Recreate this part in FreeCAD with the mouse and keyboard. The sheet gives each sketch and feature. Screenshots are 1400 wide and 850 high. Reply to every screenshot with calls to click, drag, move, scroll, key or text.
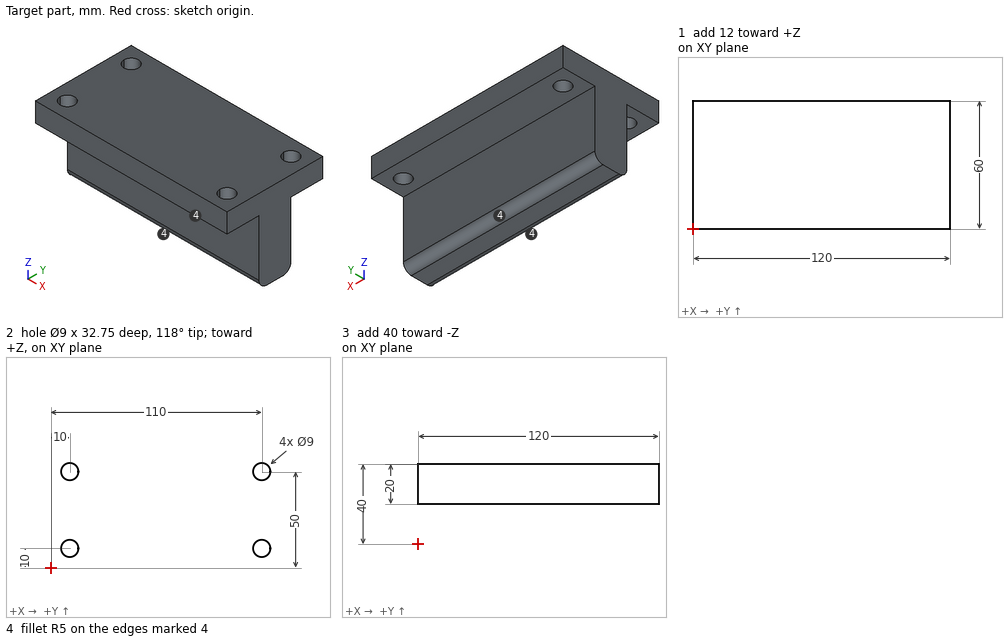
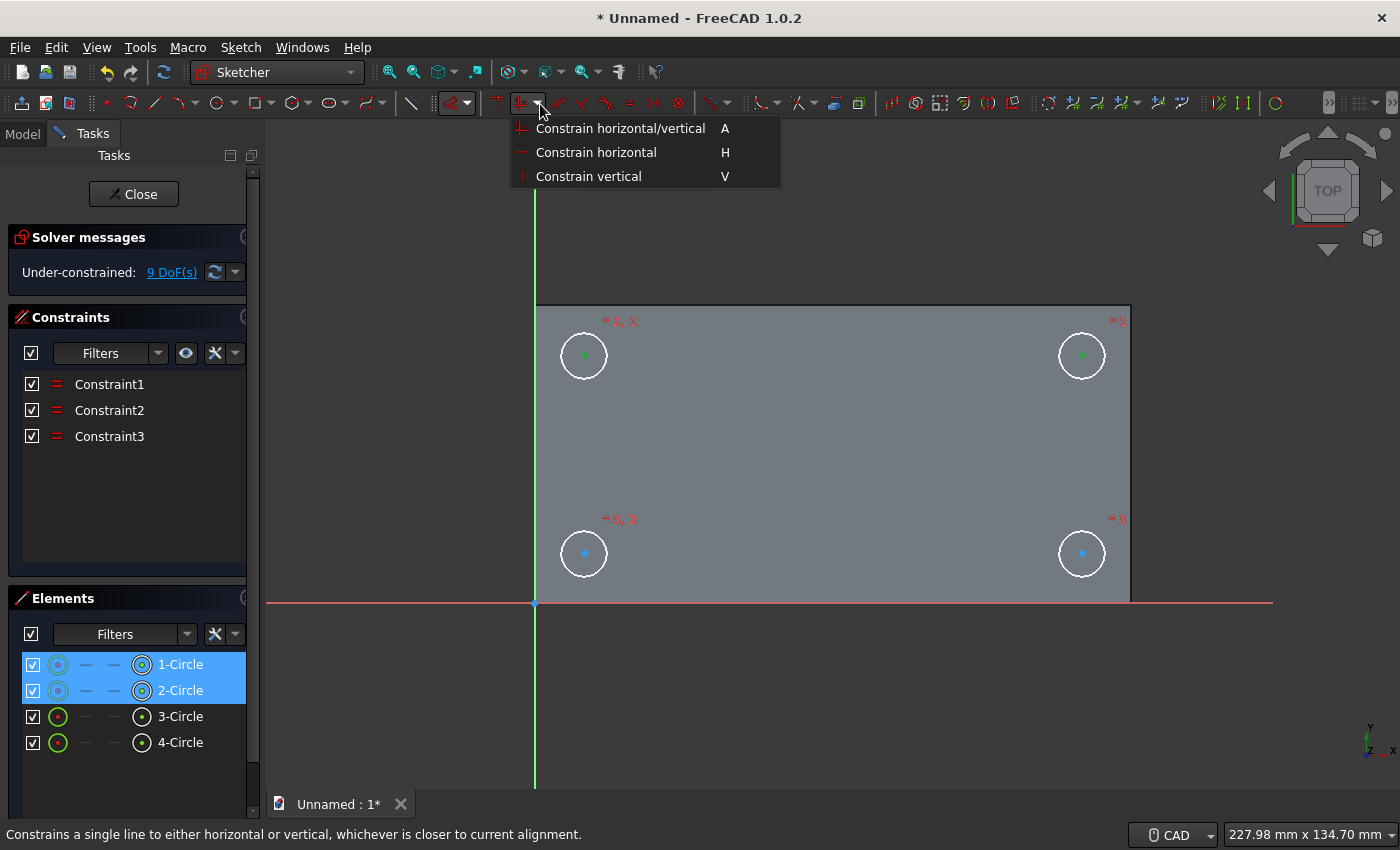
click(646, 152)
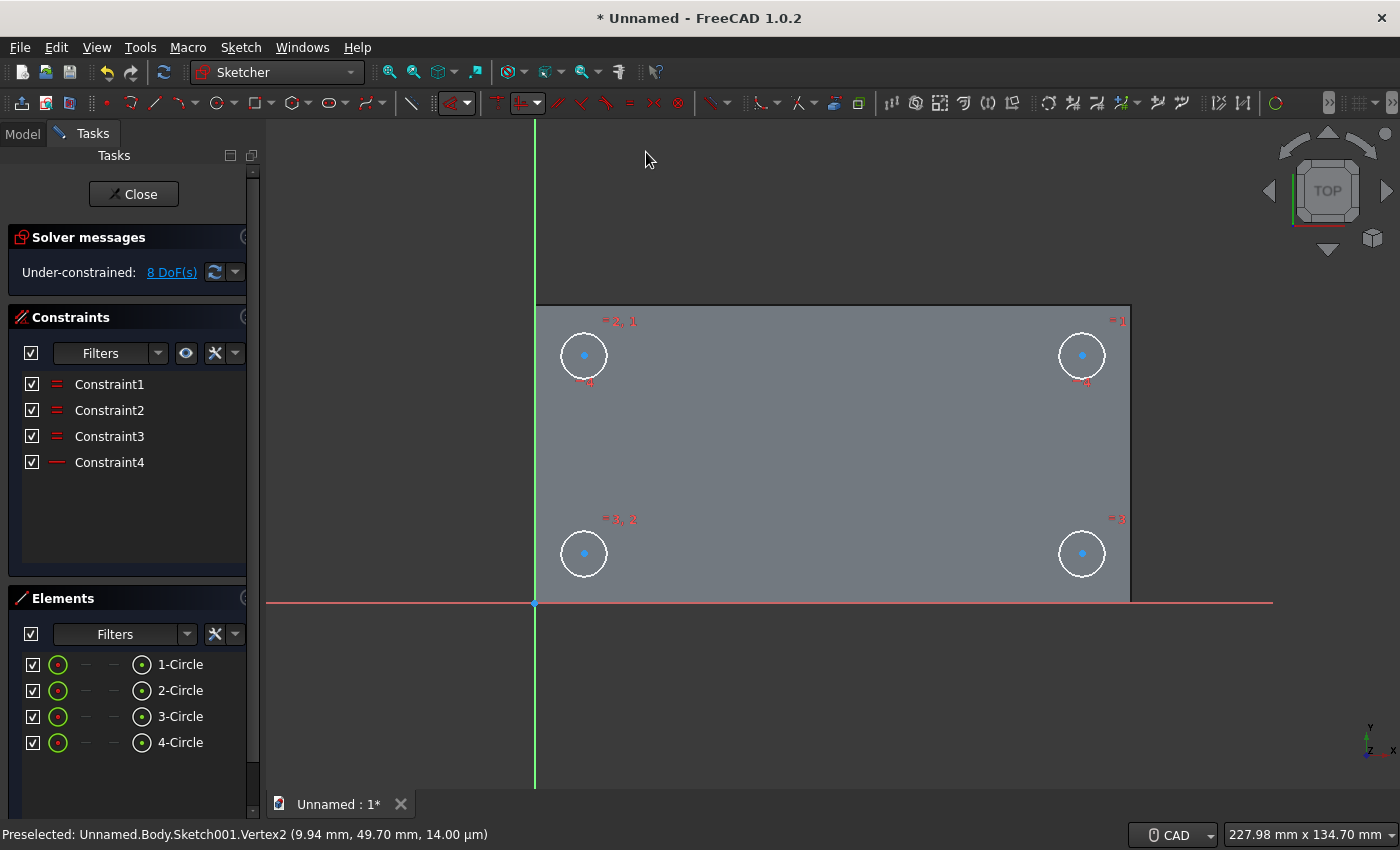
click(584, 356)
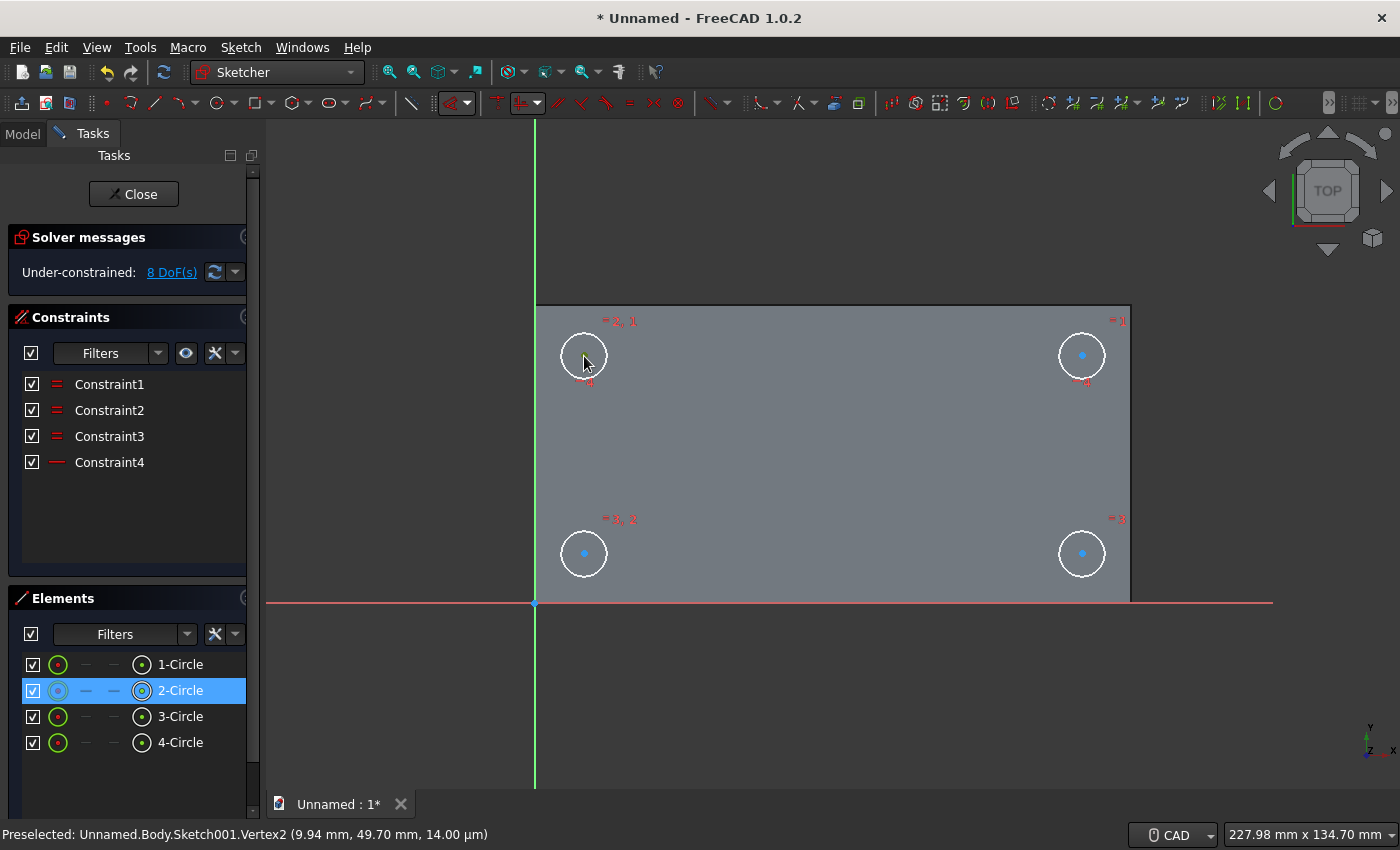
click(584, 554)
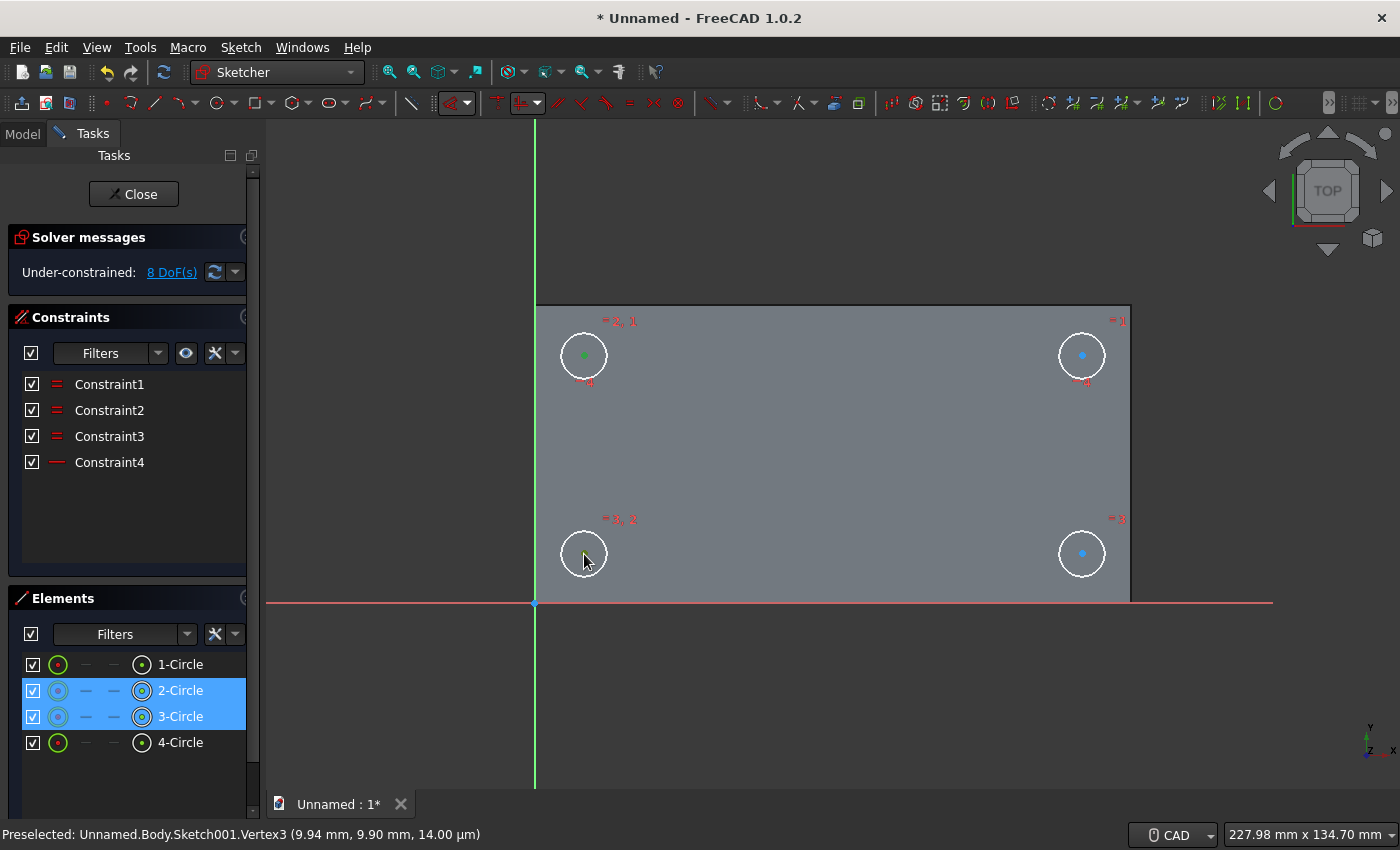
click(540, 104)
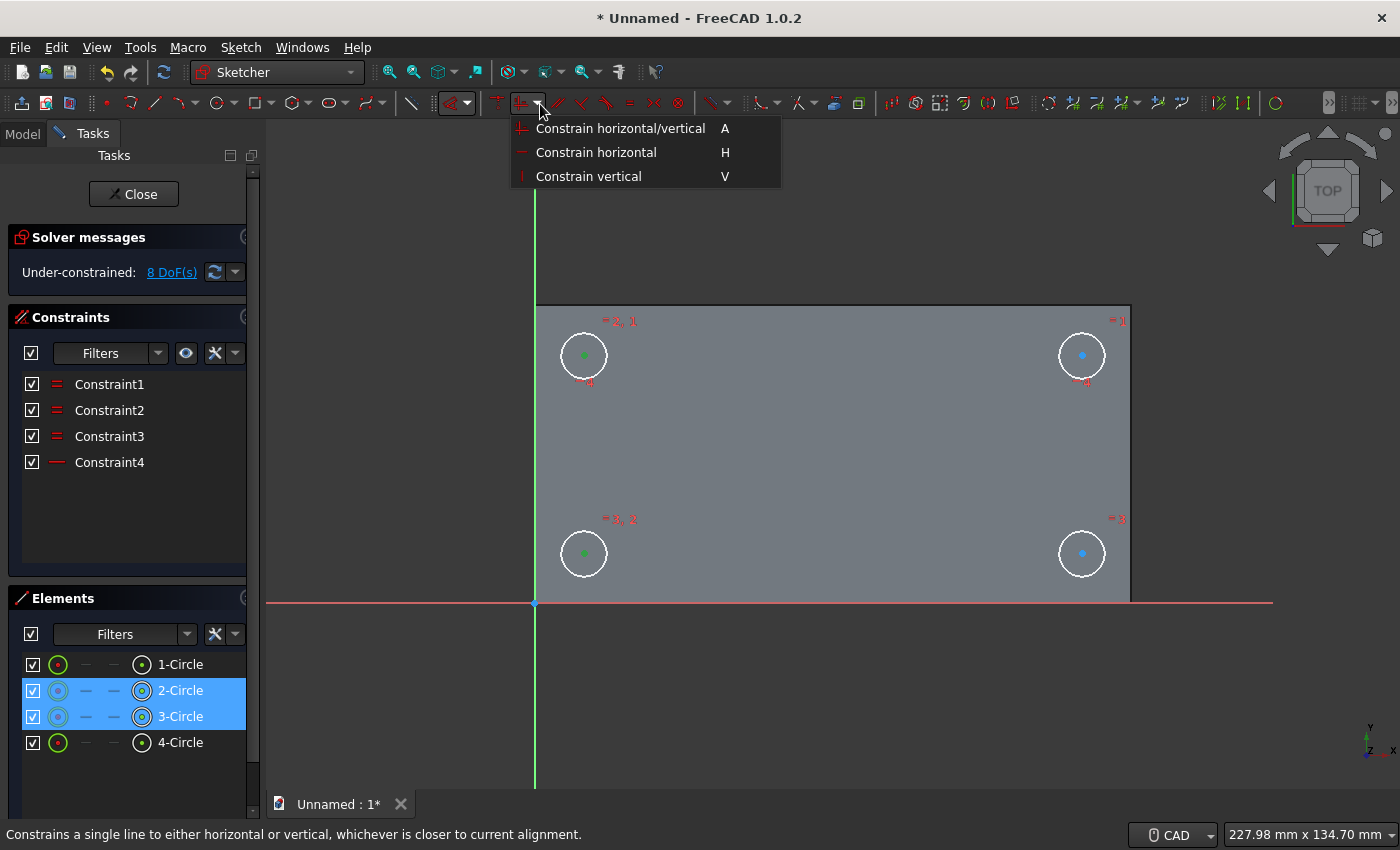
click(646, 176)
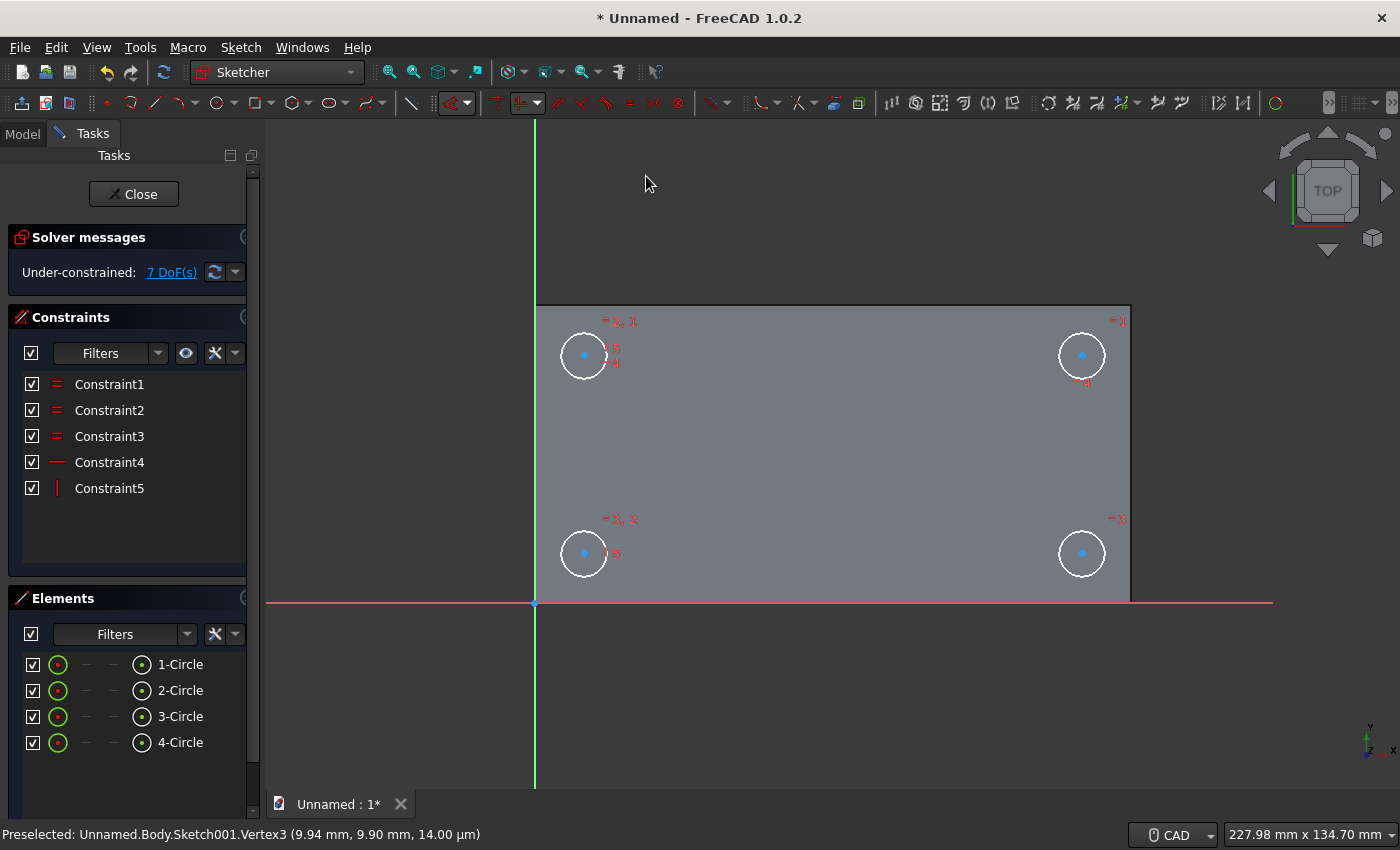
click(1082, 356)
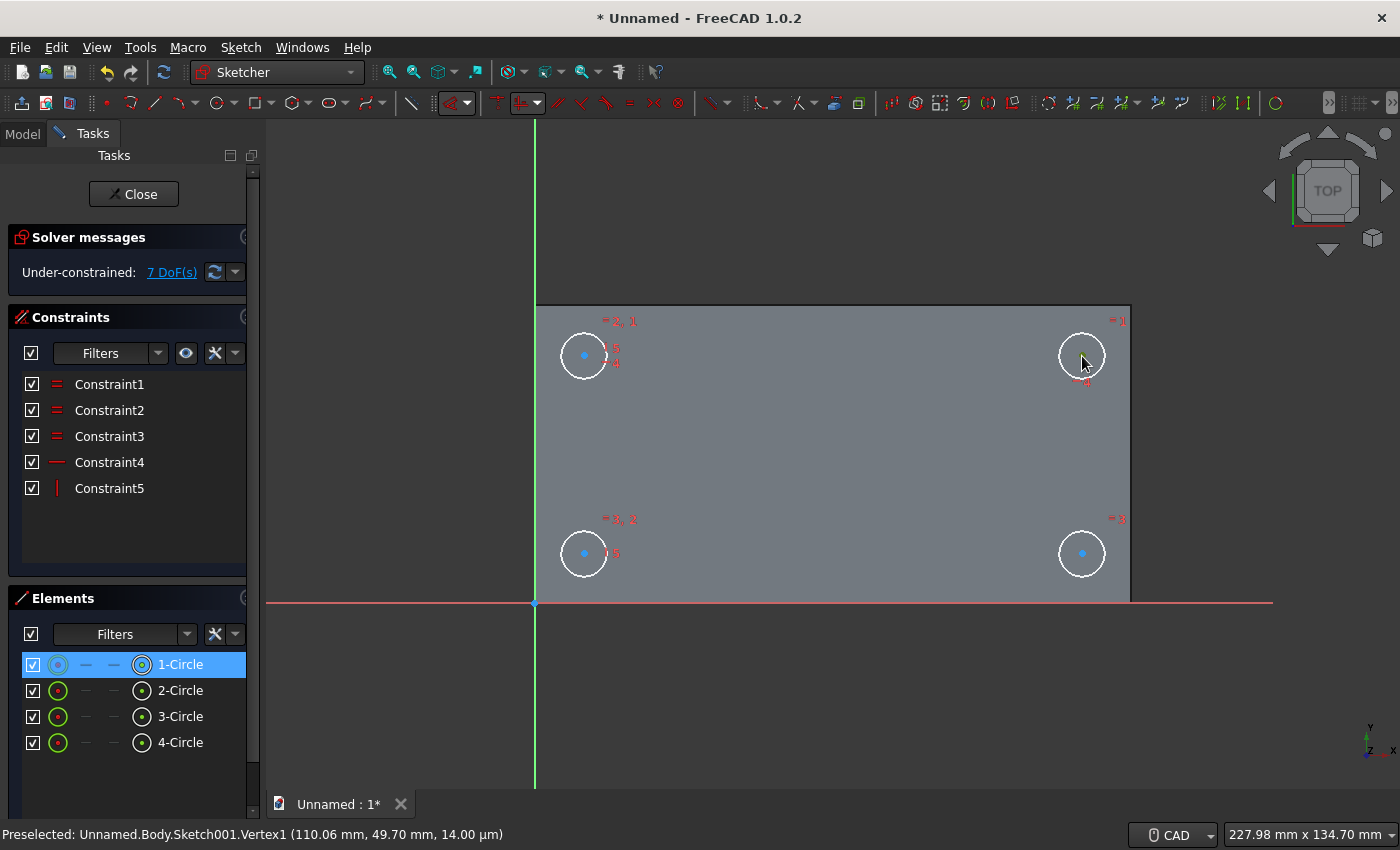
click(1082, 554)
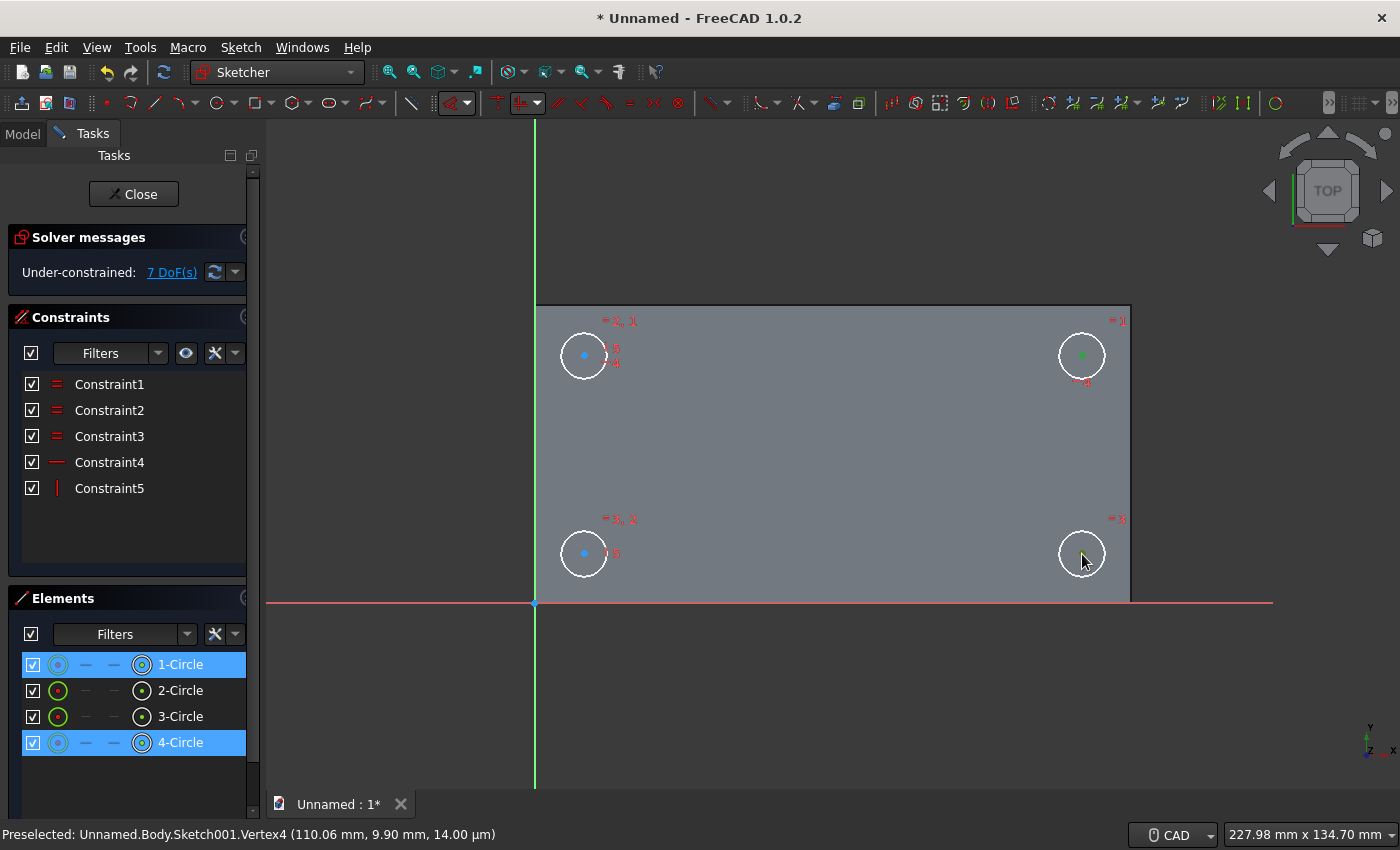
click(540, 104)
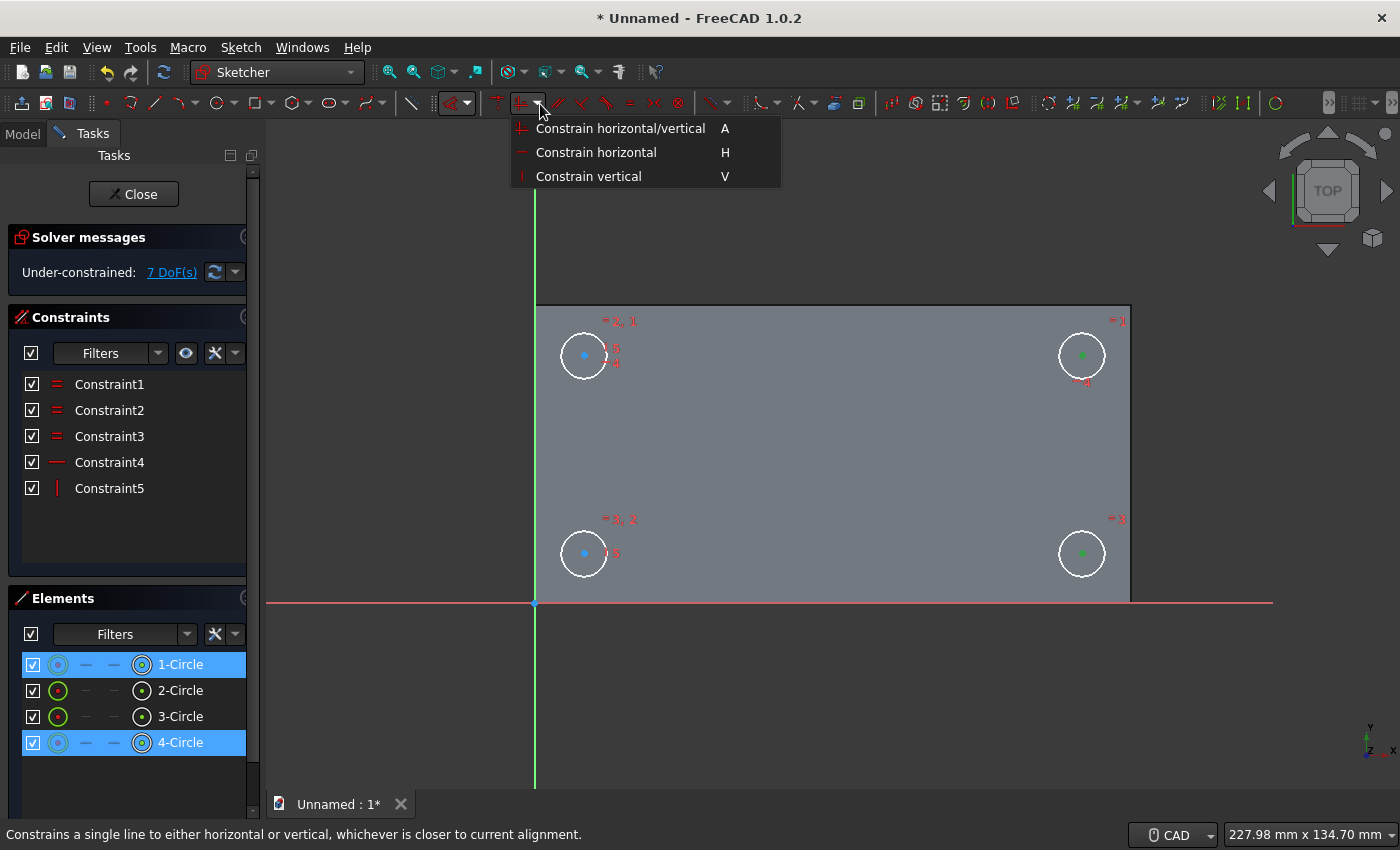
click(646, 176)